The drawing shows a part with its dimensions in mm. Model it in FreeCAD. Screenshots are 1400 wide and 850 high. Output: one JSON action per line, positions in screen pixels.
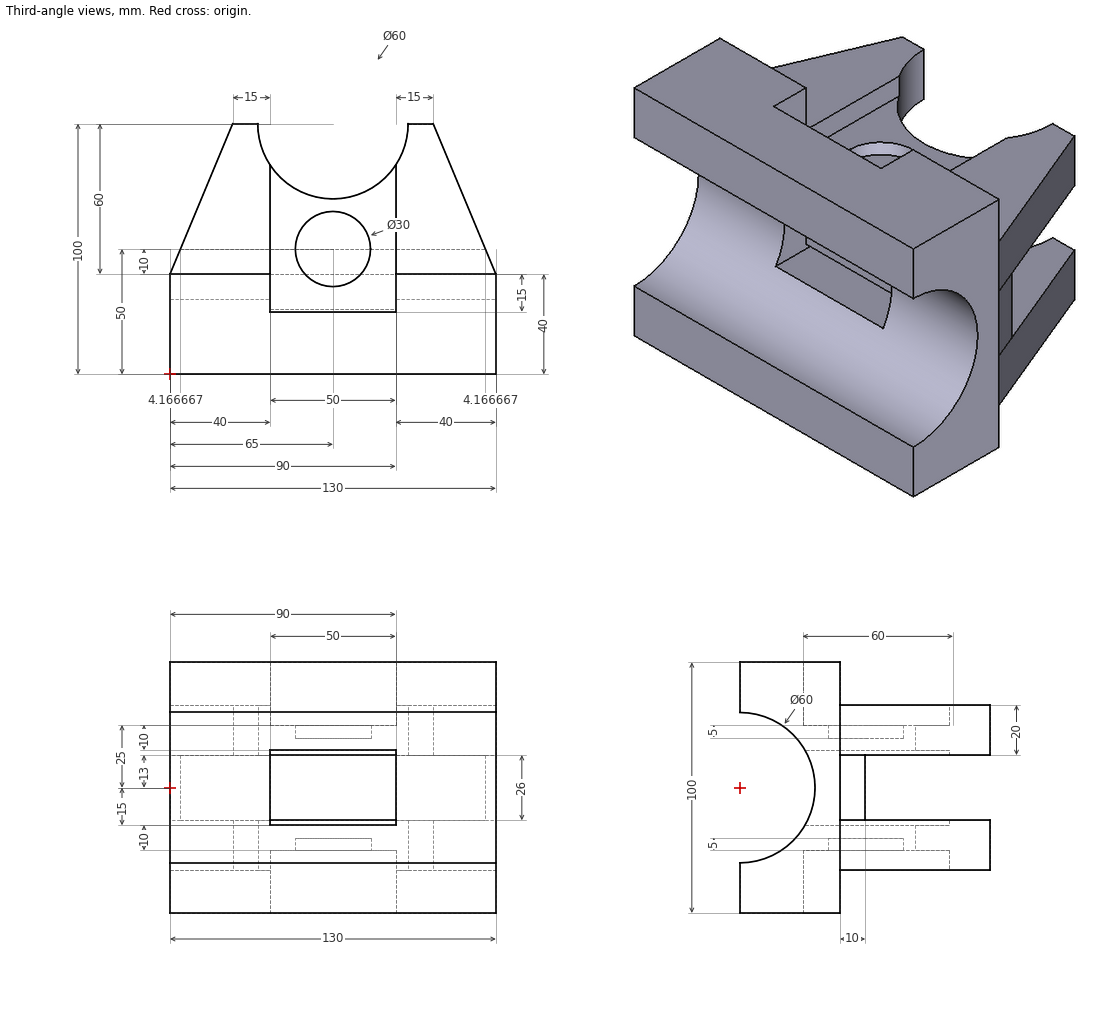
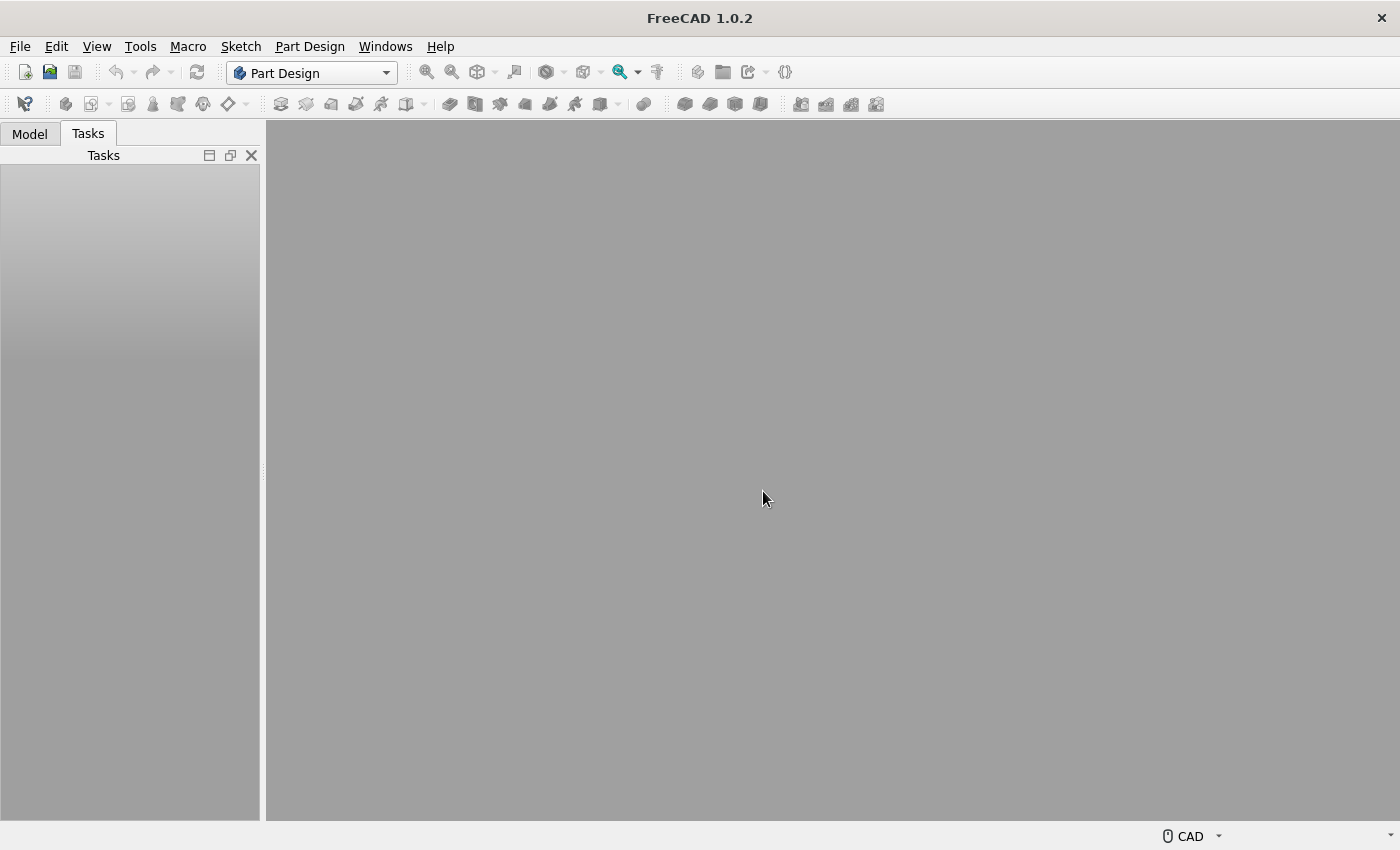
{"action": "left_click", "coordinate": [25, 72]}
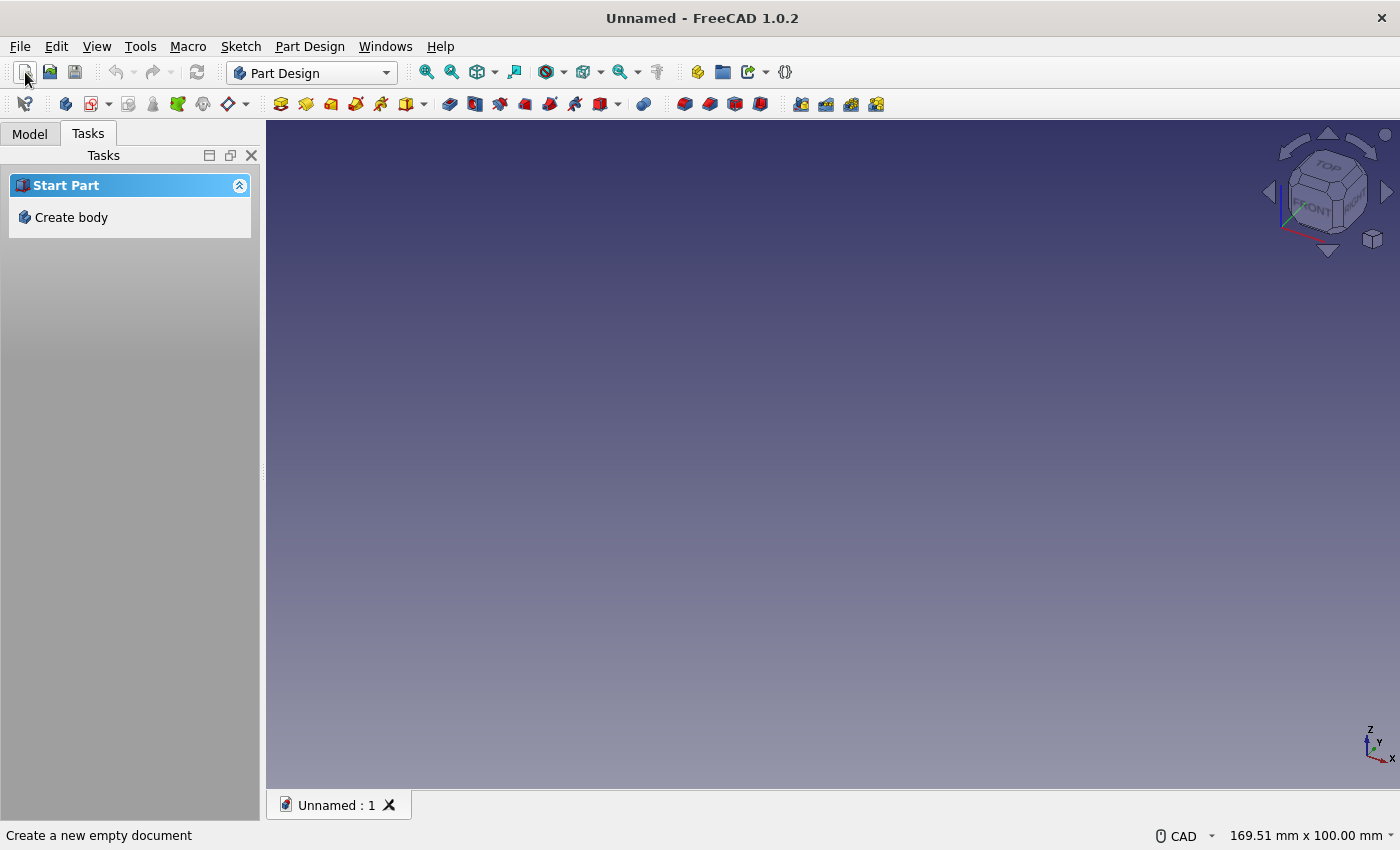
{"action": "left_click", "coordinate": [90, 104]}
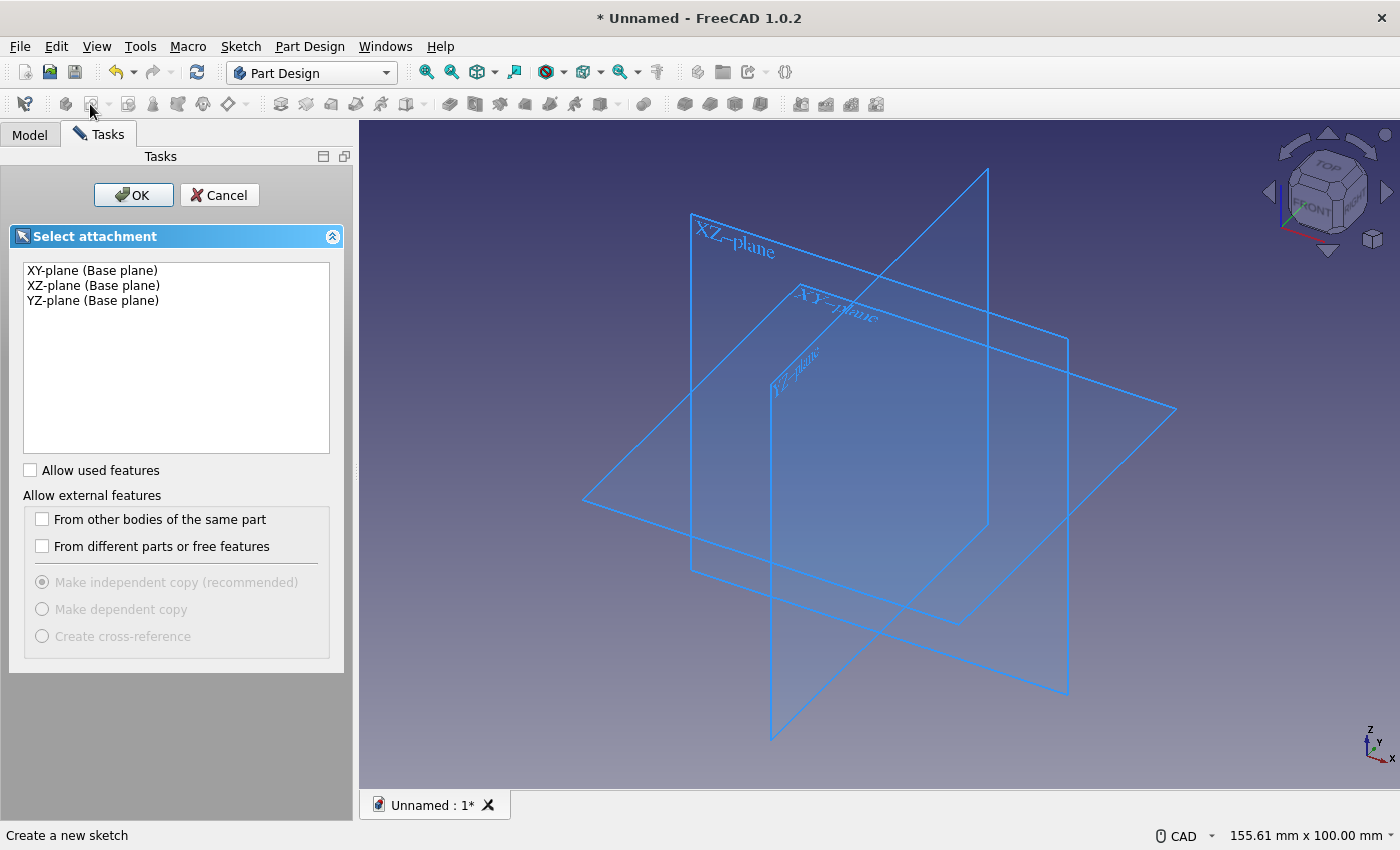
{"action": "left_click", "coordinate": [84, 270]}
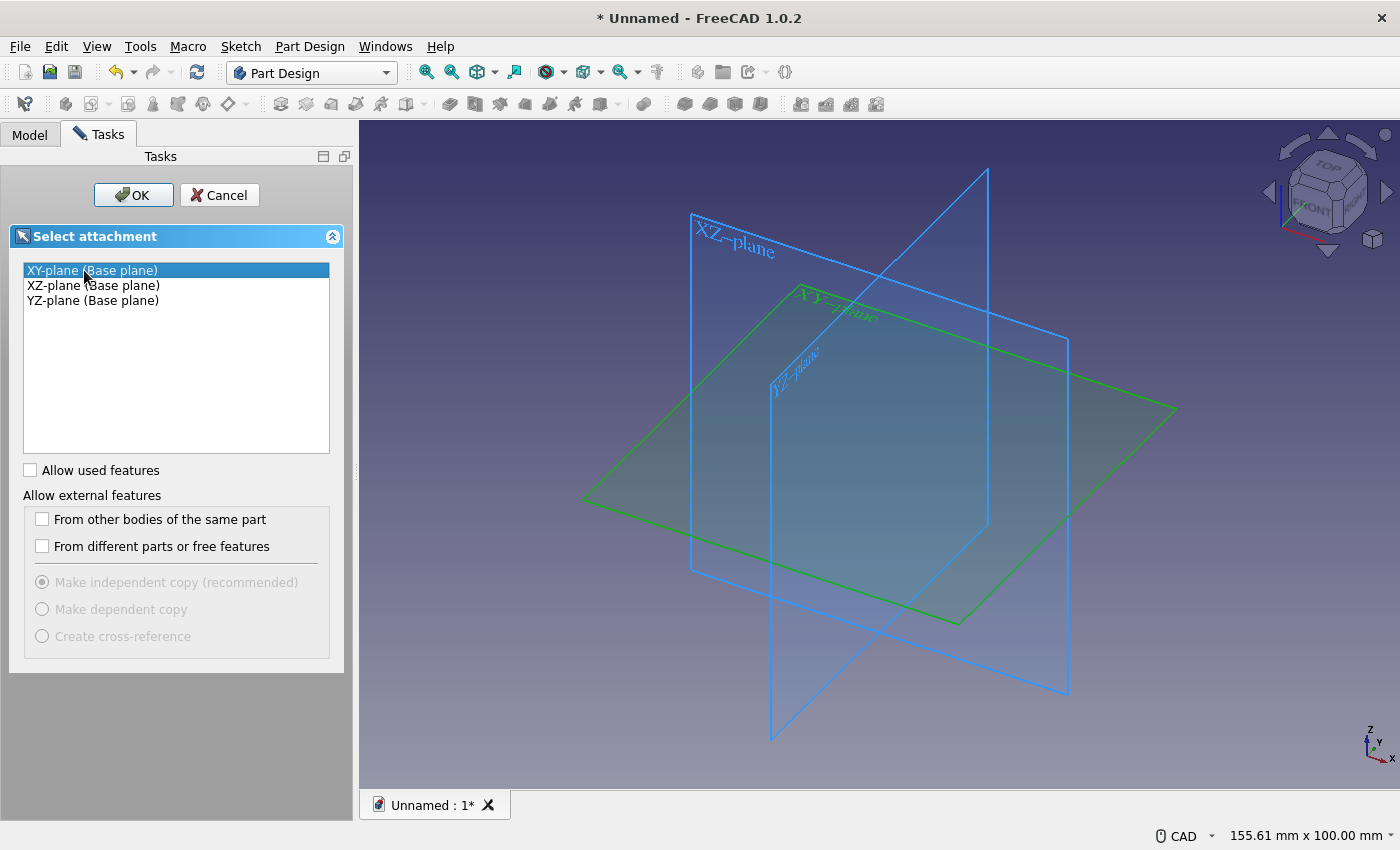
{"action": "left_click", "coordinate": [134, 195]}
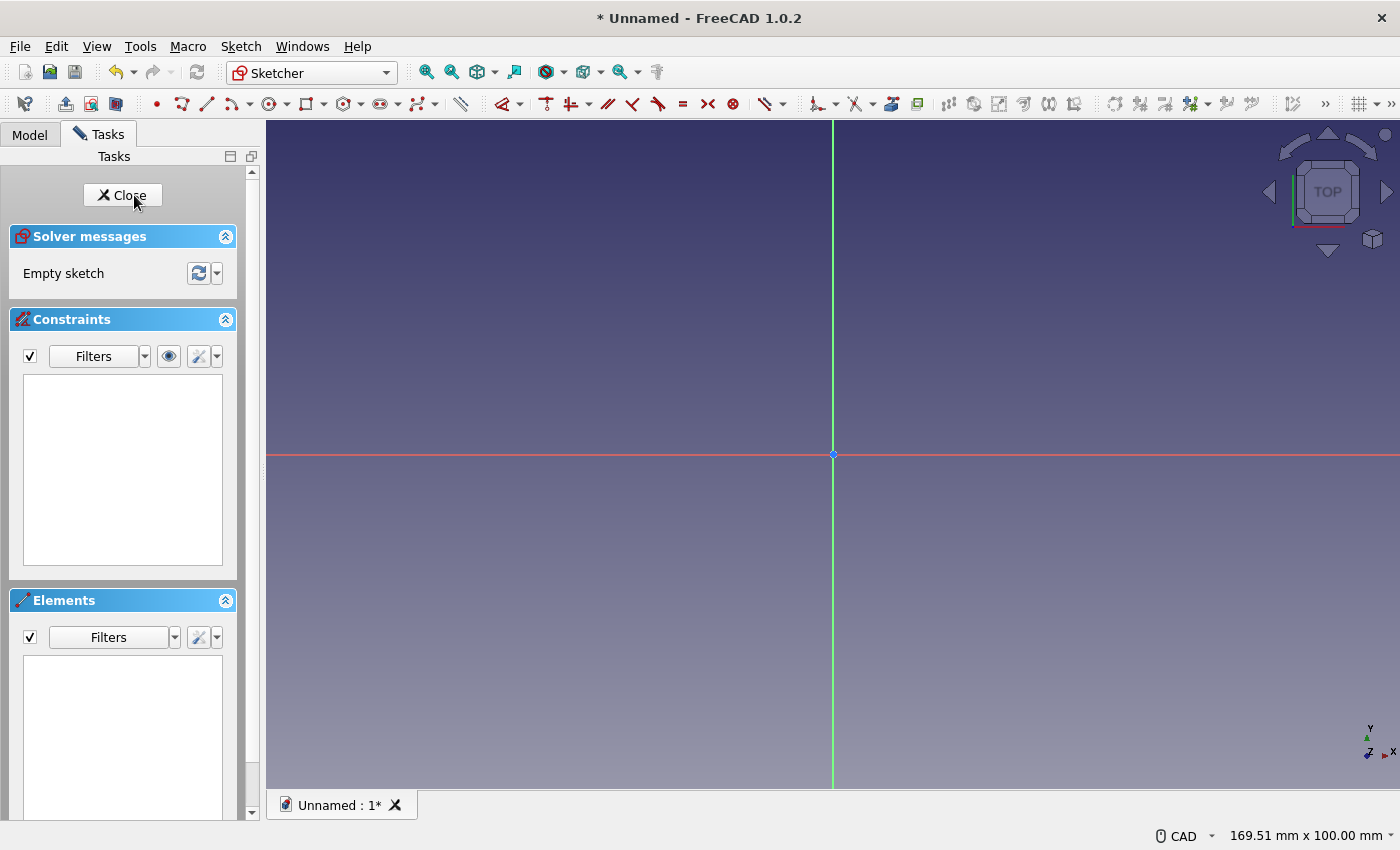
{"action": "scroll", "coordinate": [294, 617], "scroll_direction": "down", "scroll_amount": 3}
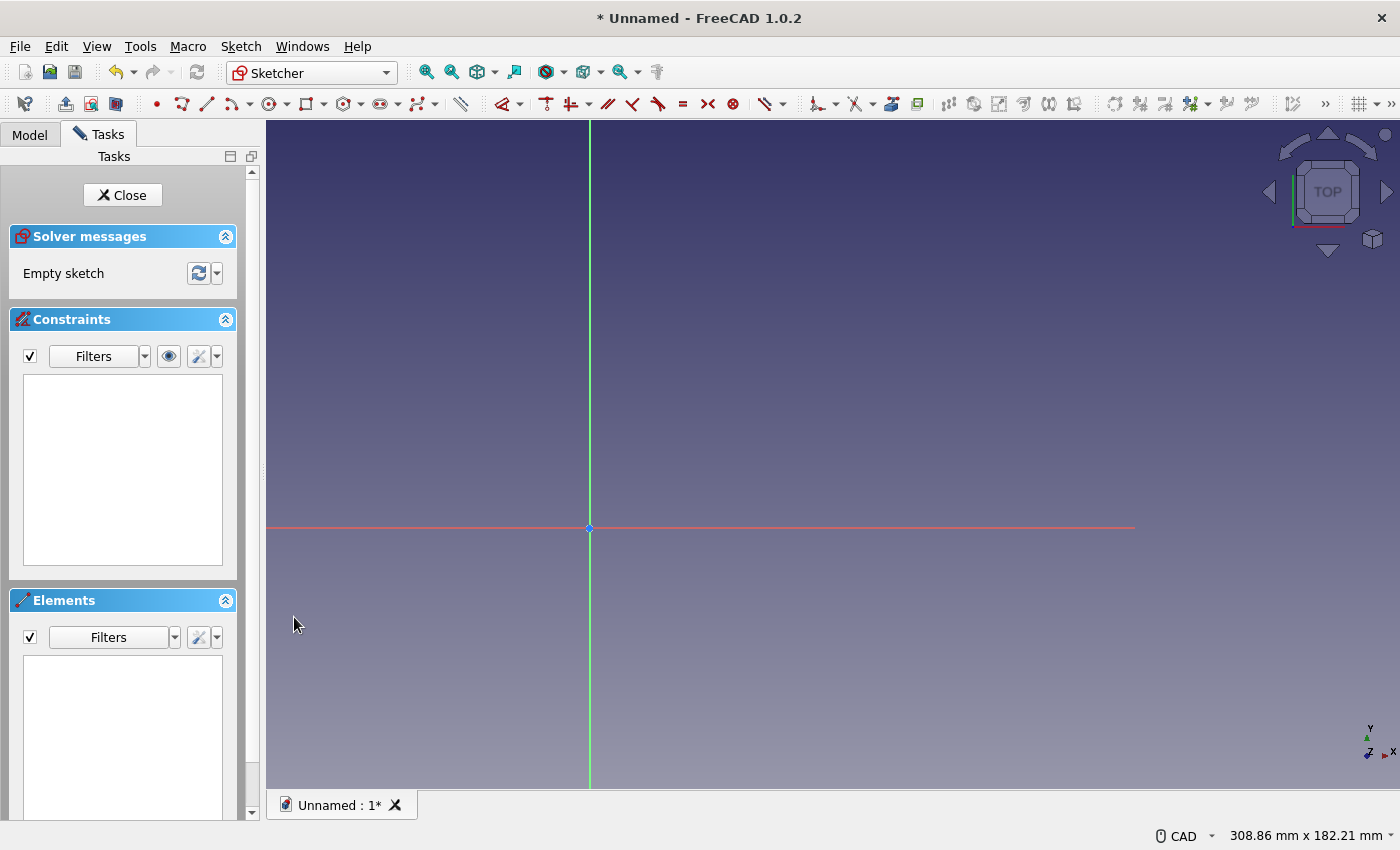
{"action": "scroll", "coordinate": [959, 455], "scroll_direction": "up", "scroll_amount": 2}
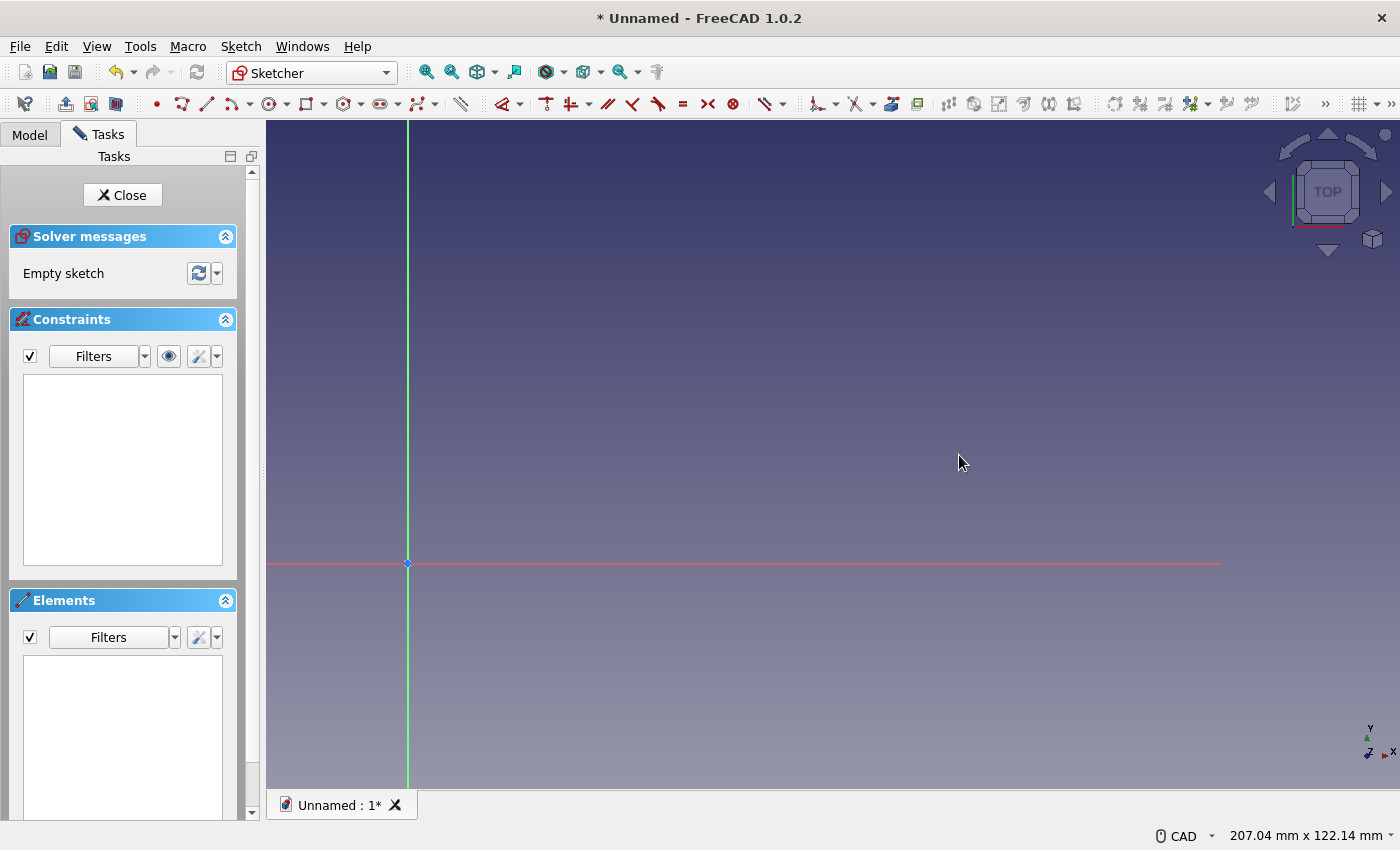
{"action": "left_click", "coordinate": [182, 104]}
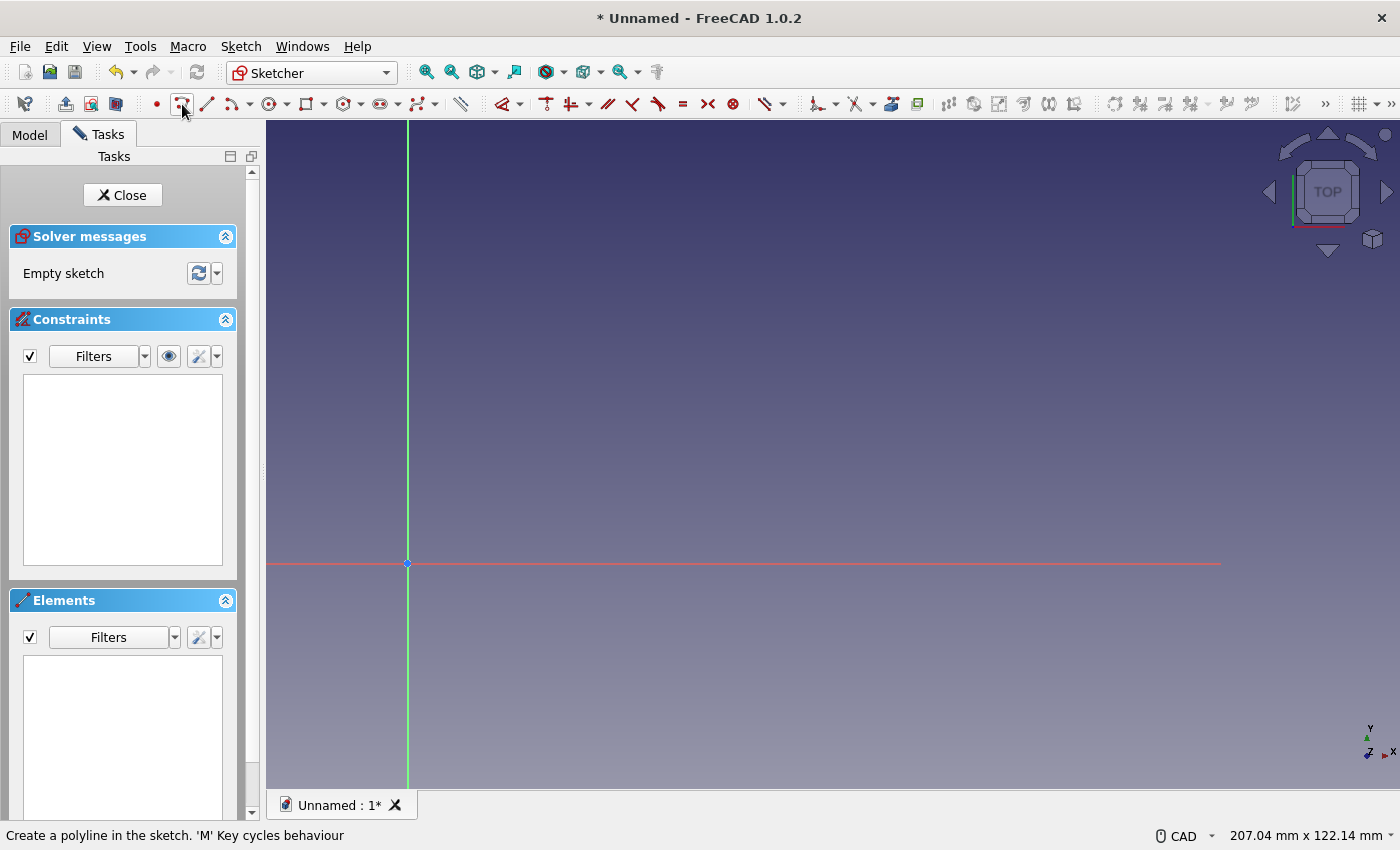
{"action": "left_click", "coordinate": [408, 564]}
{"action": "left_click", "coordinate": [1120, 555]}
{"action": "left_click", "coordinate": [1120, 345]}
{"action": "left_click", "coordinate": [901, 345]}
{"action": "left_click", "coordinate": [901, 427]}
{"action": "left_click", "coordinate": [627, 427]}
{"action": "left_click", "coordinate": [627, 345]}
{"action": "left_click", "coordinate": [417, 345]}
{"action": "left_click", "coordinate": [408, 564]}
{"action": "key", "text": "Escape"}
{"action": "key", "text": "Escape"}